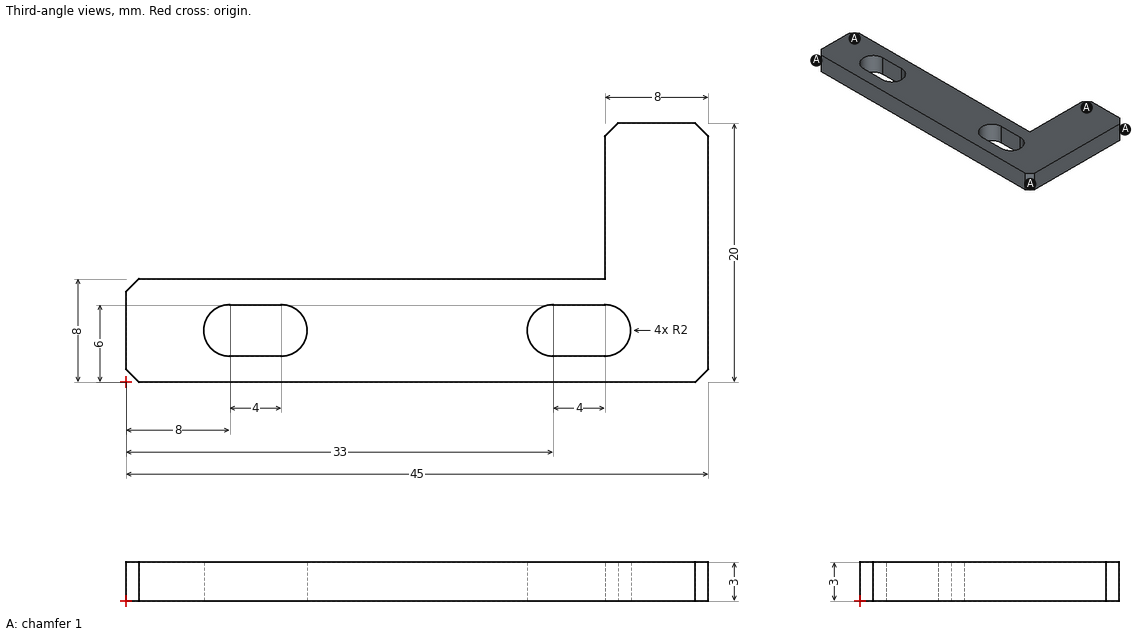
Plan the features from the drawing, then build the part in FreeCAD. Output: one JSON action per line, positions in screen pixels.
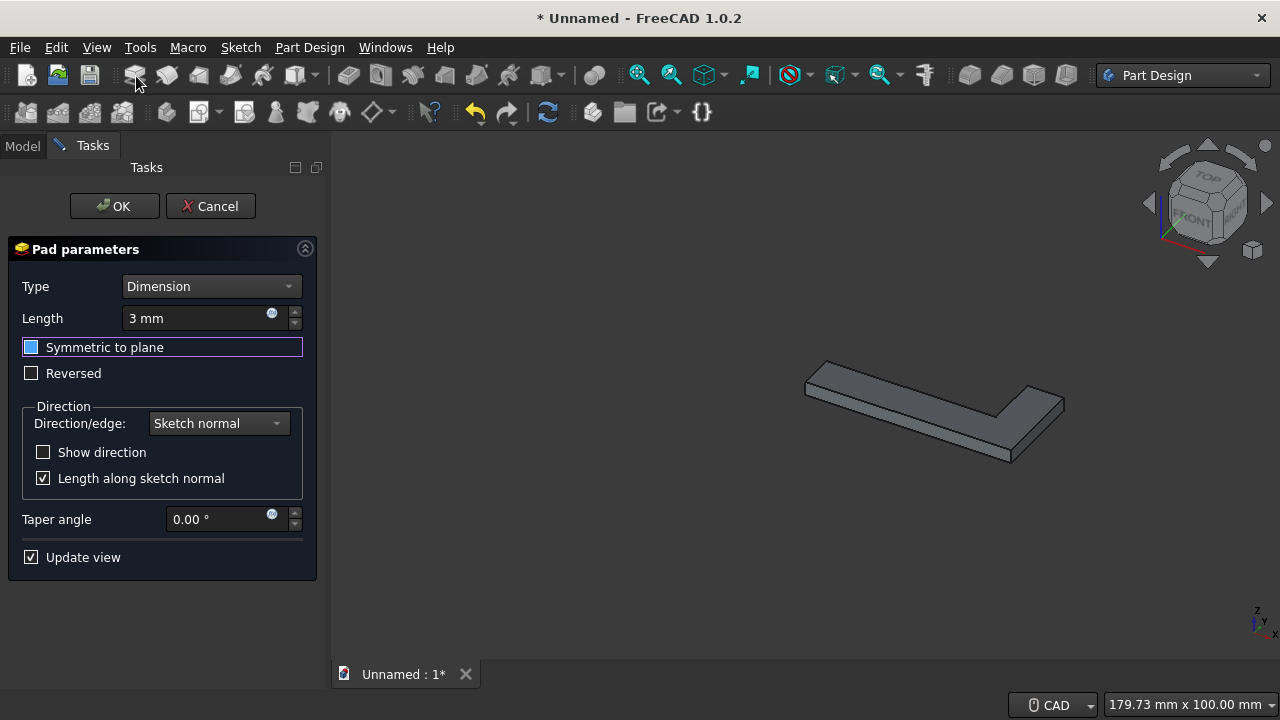
{"action": "left_click", "coordinate": [115, 206]}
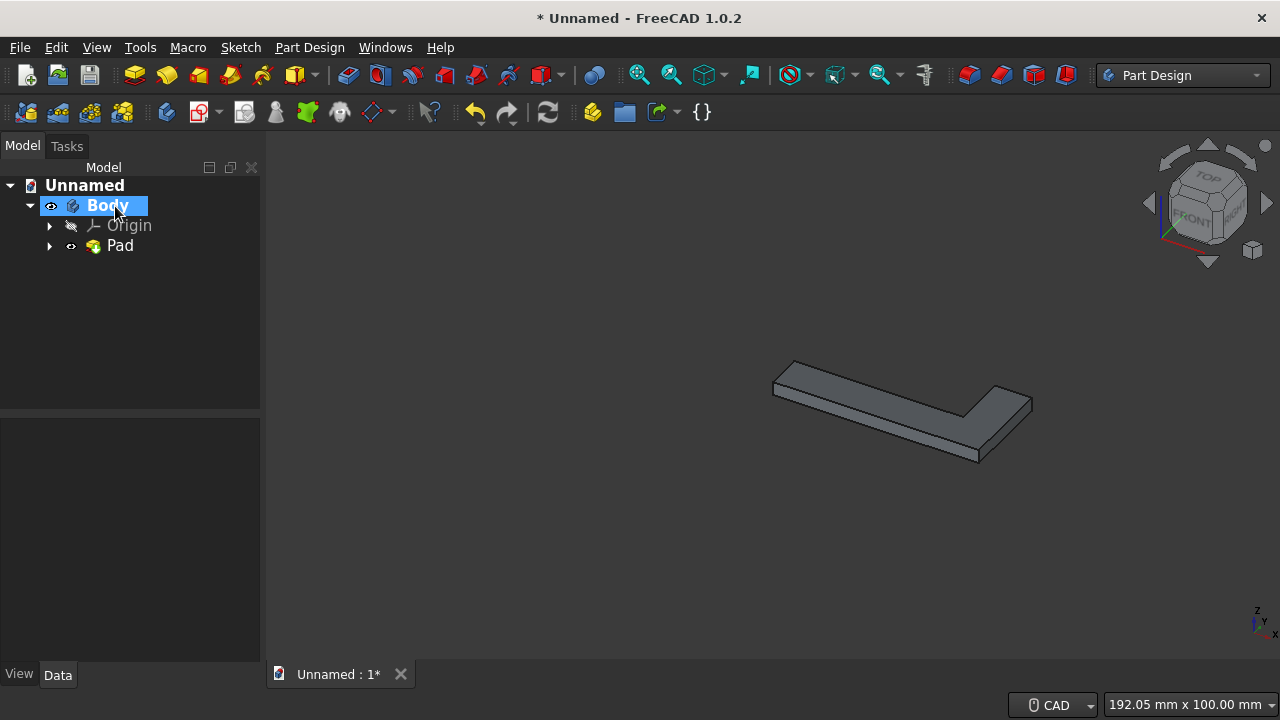
{"action": "left_click", "coordinate": [640, 76]}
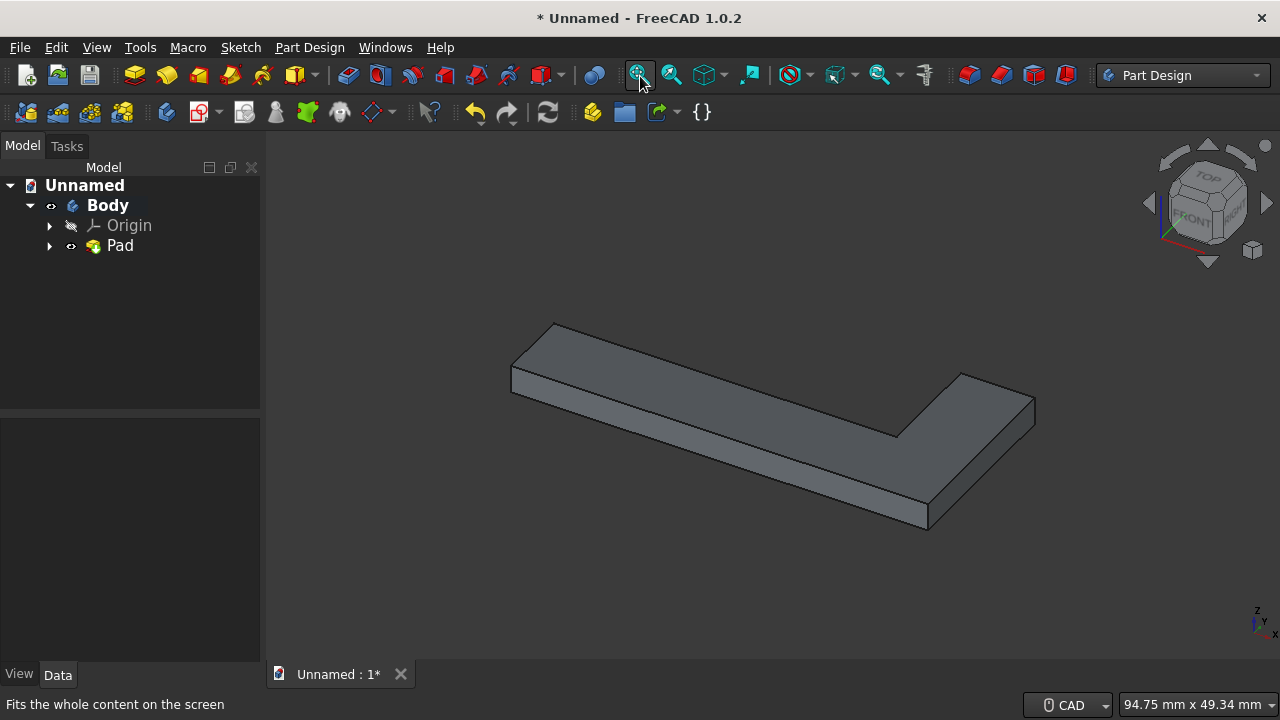
{"action": "left_click", "coordinate": [200, 112]}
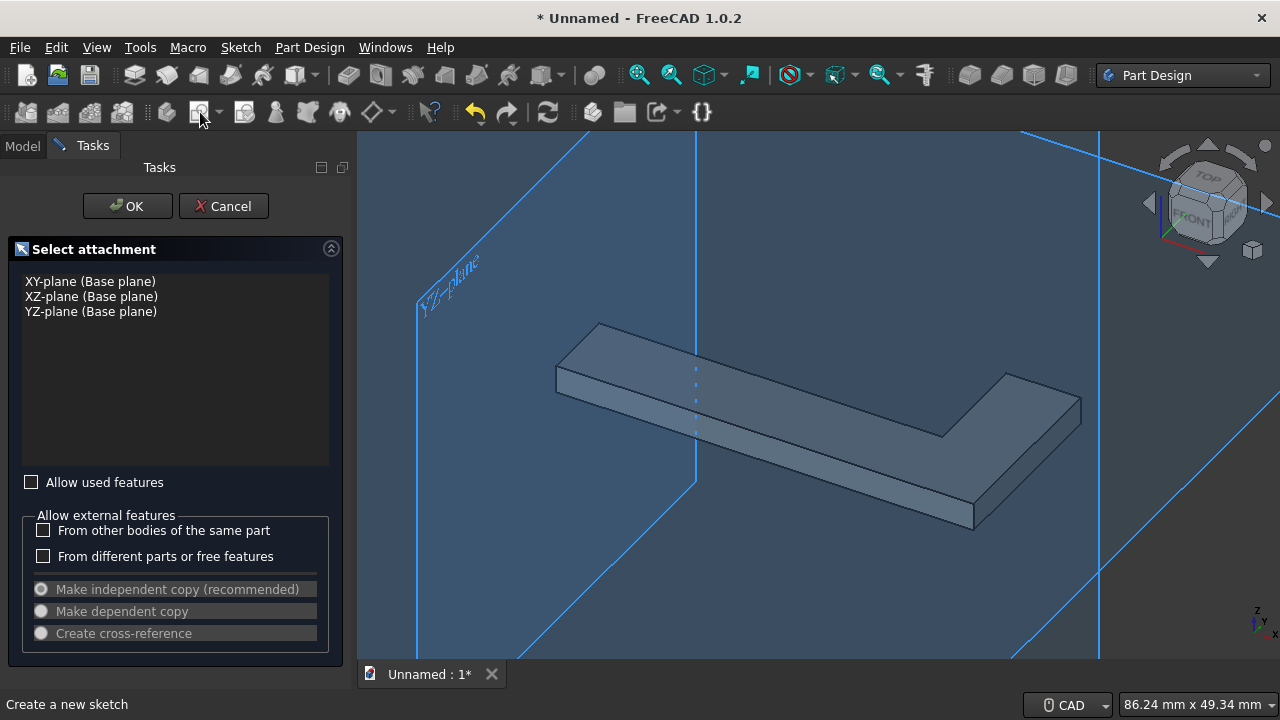
{"action": "left_click", "coordinate": [82, 282]}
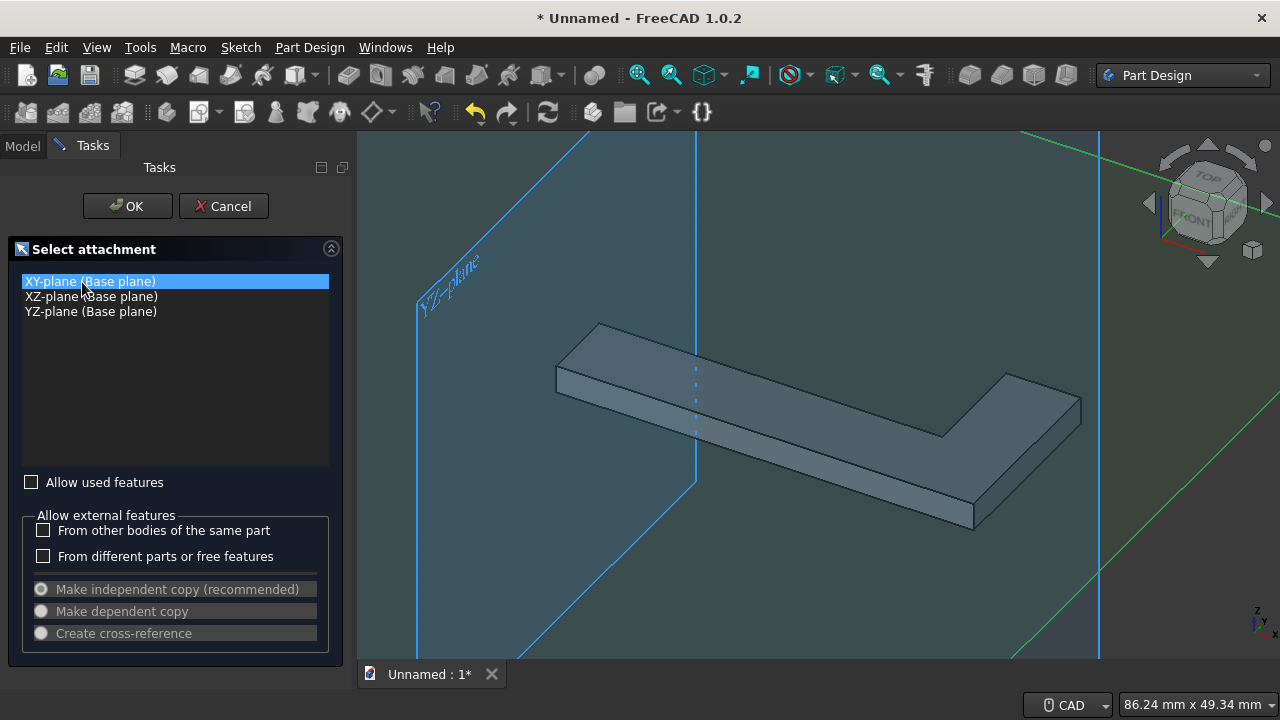
{"action": "left_click", "coordinate": [128, 206]}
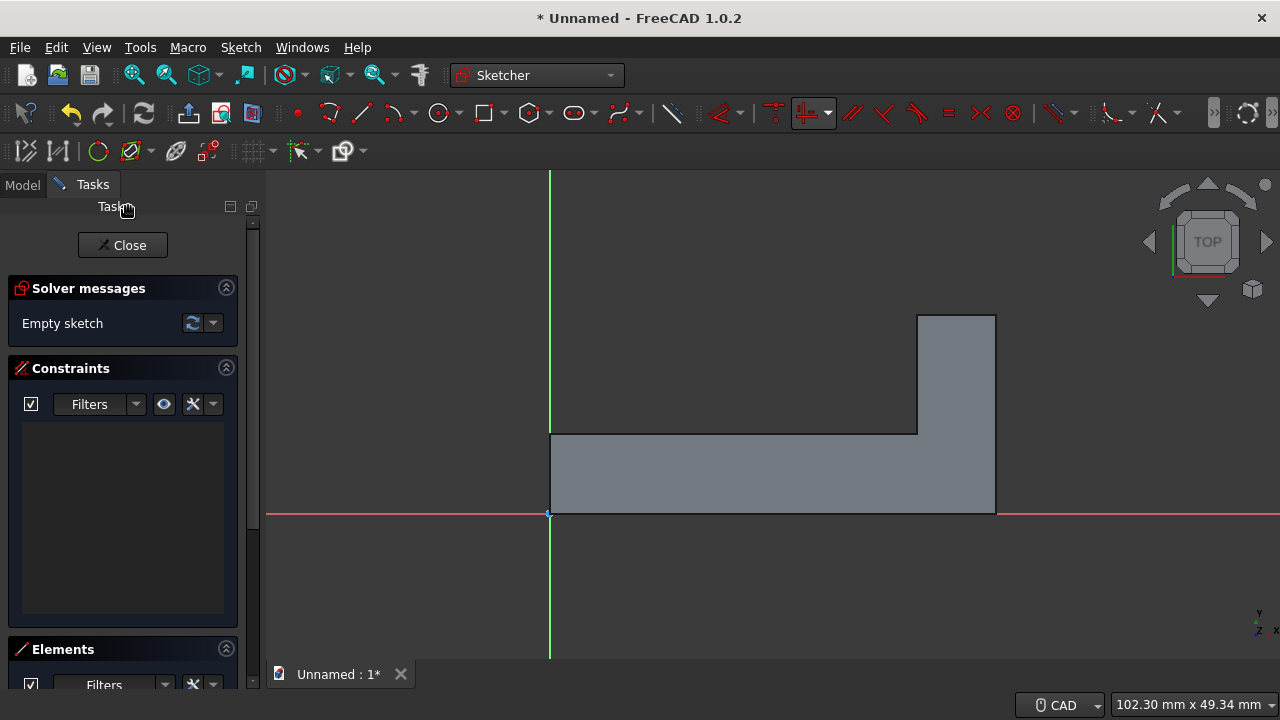
{"action": "key", "text": "q s"}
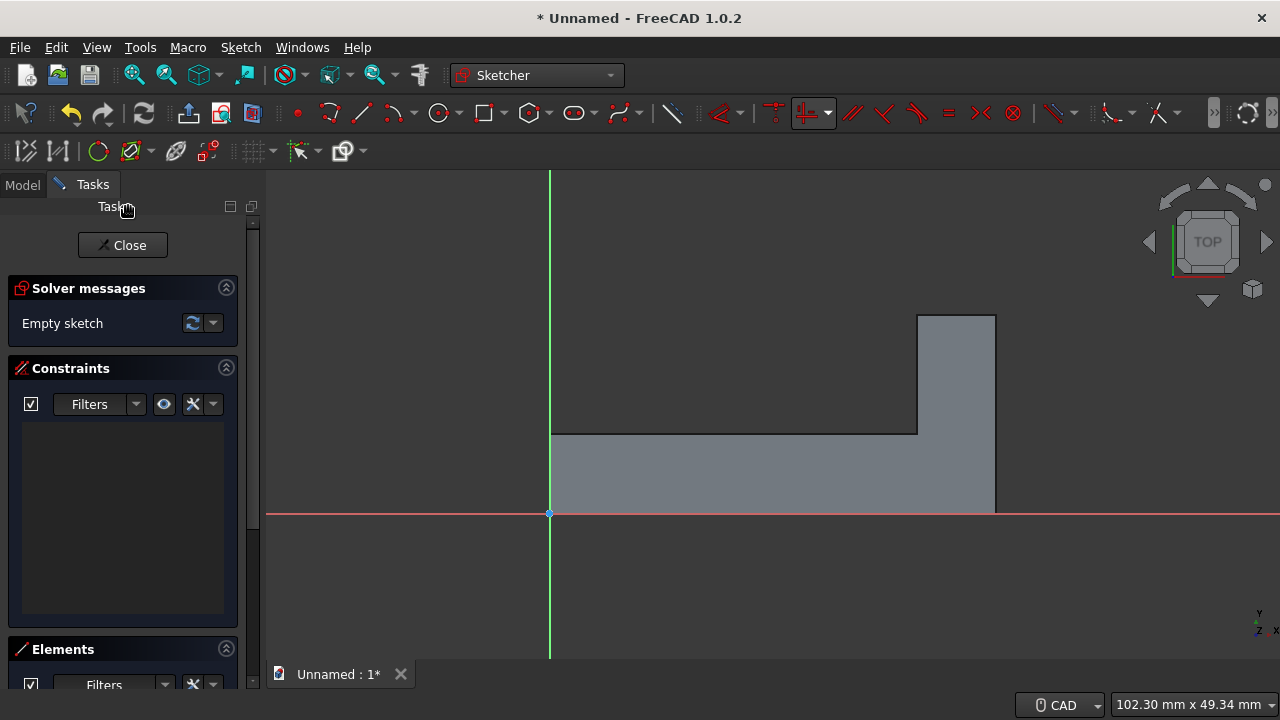
{"action": "scroll", "coordinate": [822, 625], "scroll_direction": "up", "scroll_amount": 2}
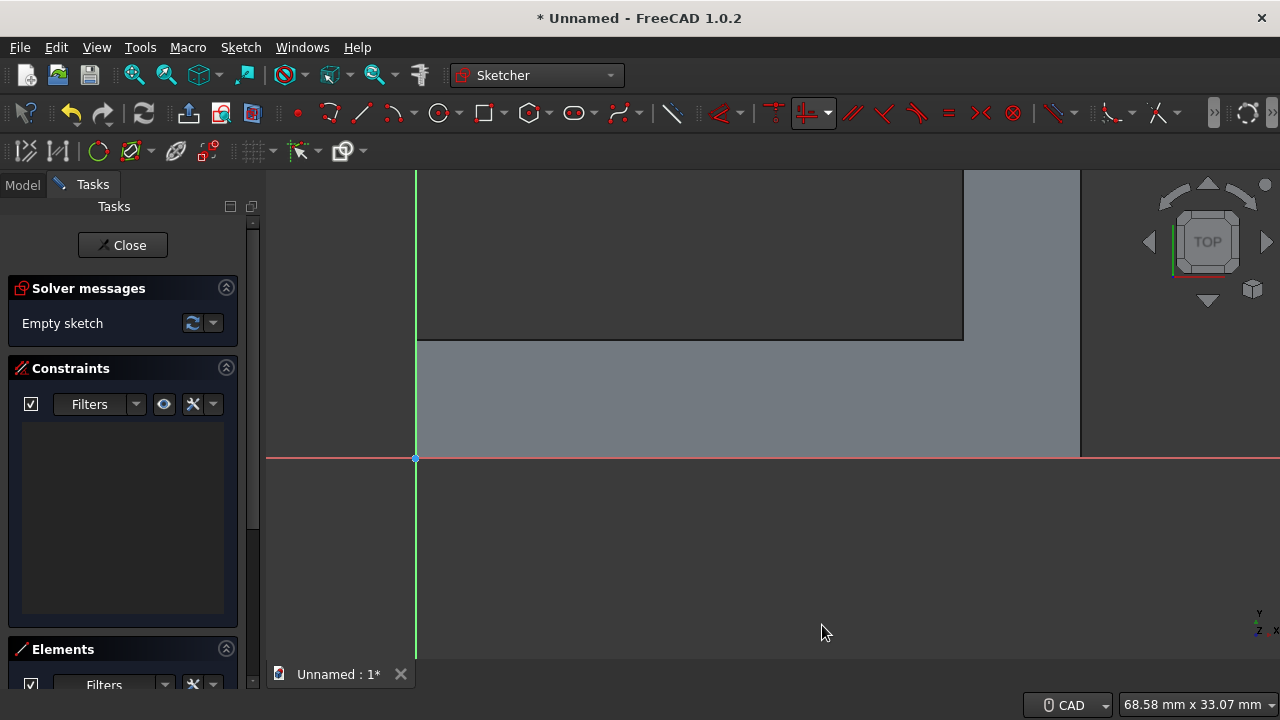
{"action": "left_click", "coordinate": [574, 114]}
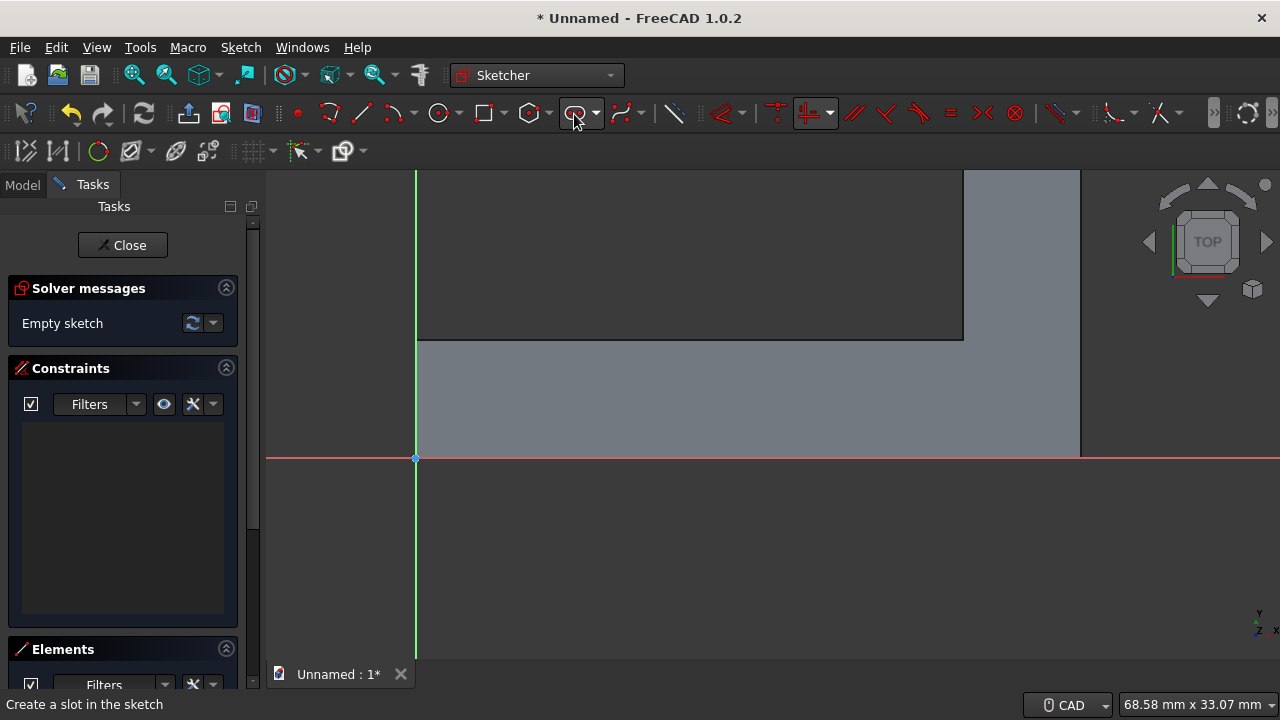
{"action": "left_click", "coordinate": [904, 399]}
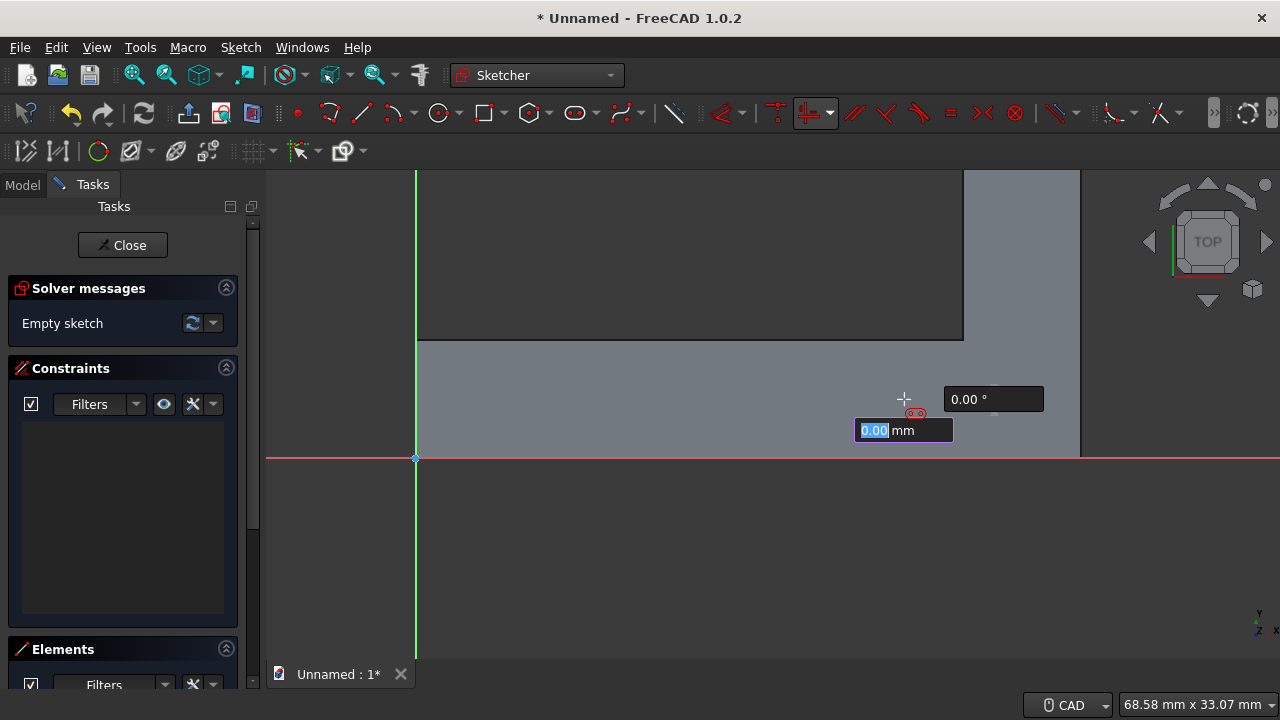
{"action": "left_click", "coordinate": [963, 399]}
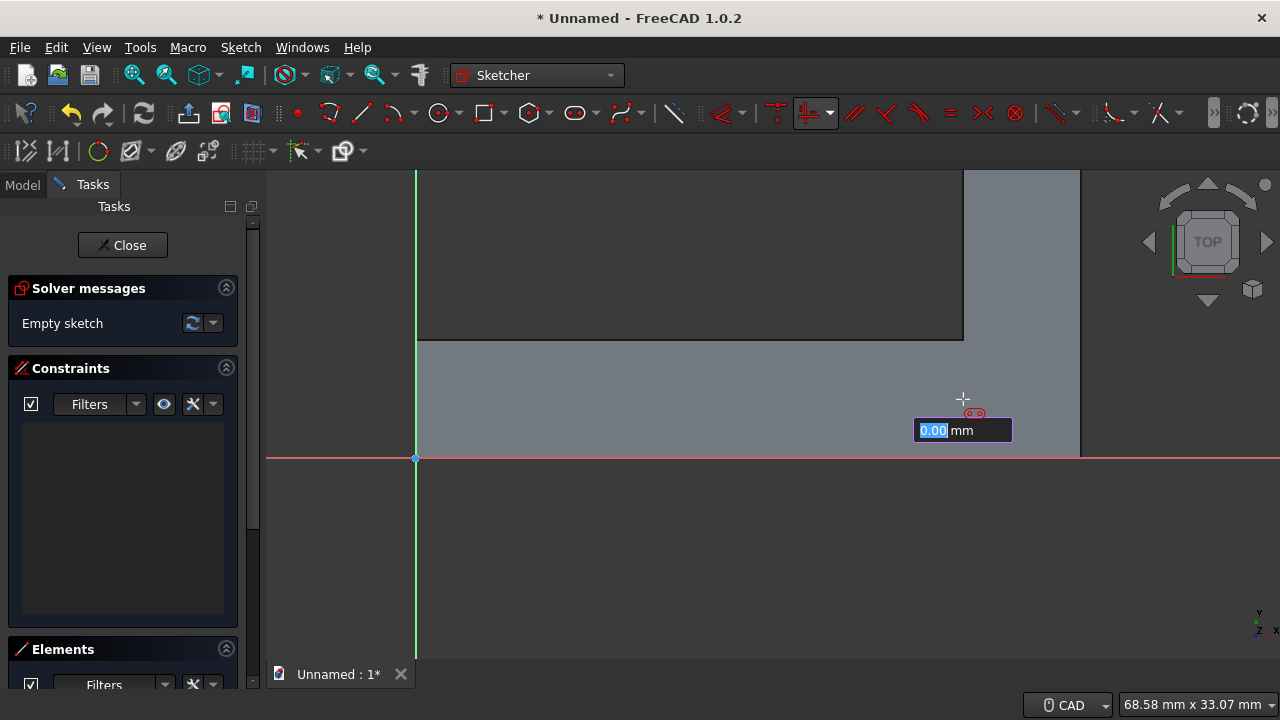
{"action": "left_click", "coordinate": [933, 370]}